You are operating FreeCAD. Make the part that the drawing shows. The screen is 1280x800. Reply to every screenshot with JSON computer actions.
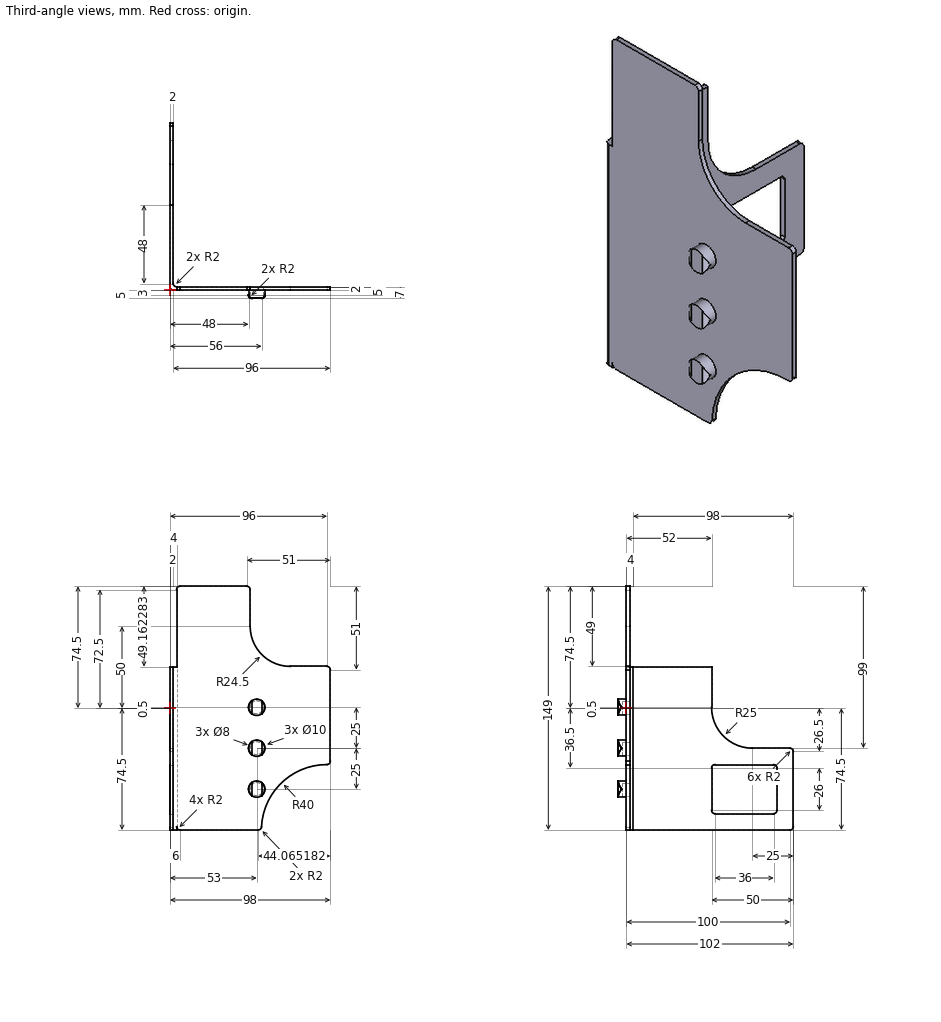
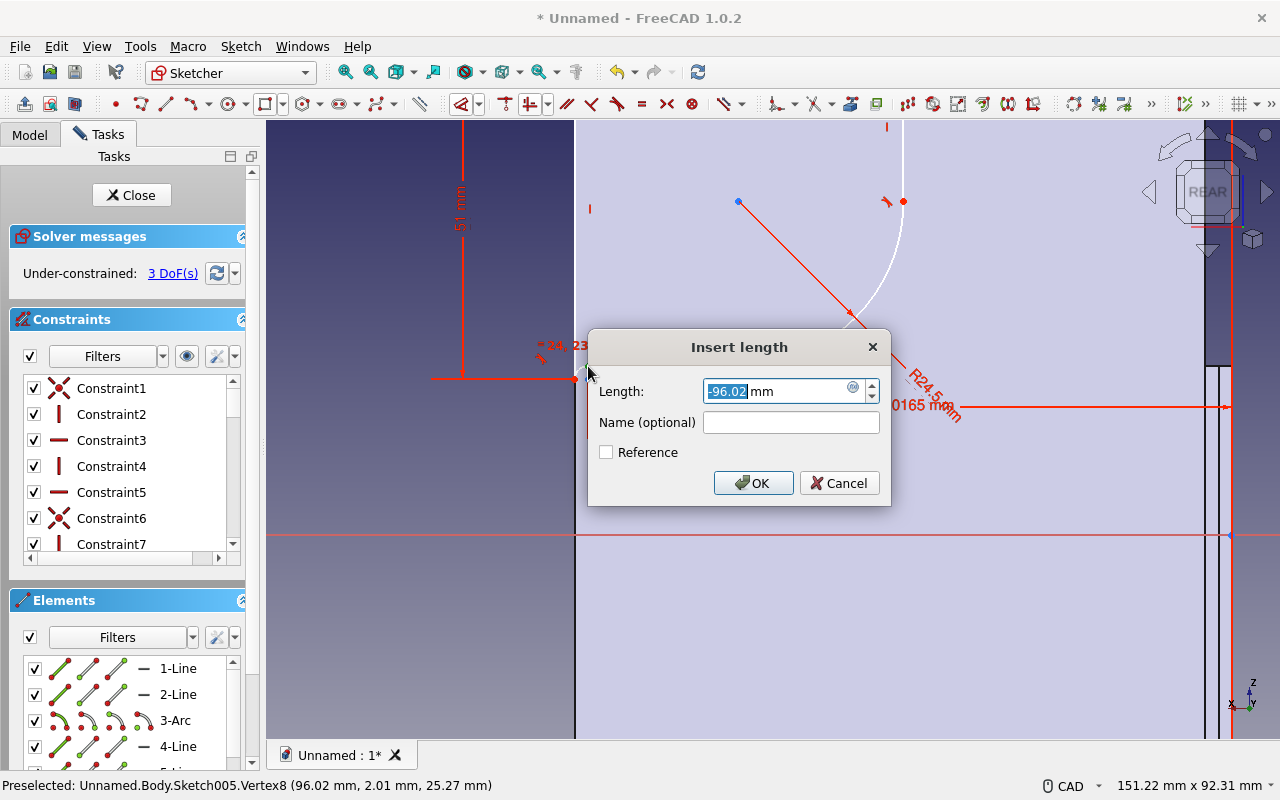
{"action": "type", "text": "-96"}
{"action": "key", "text": "Return"}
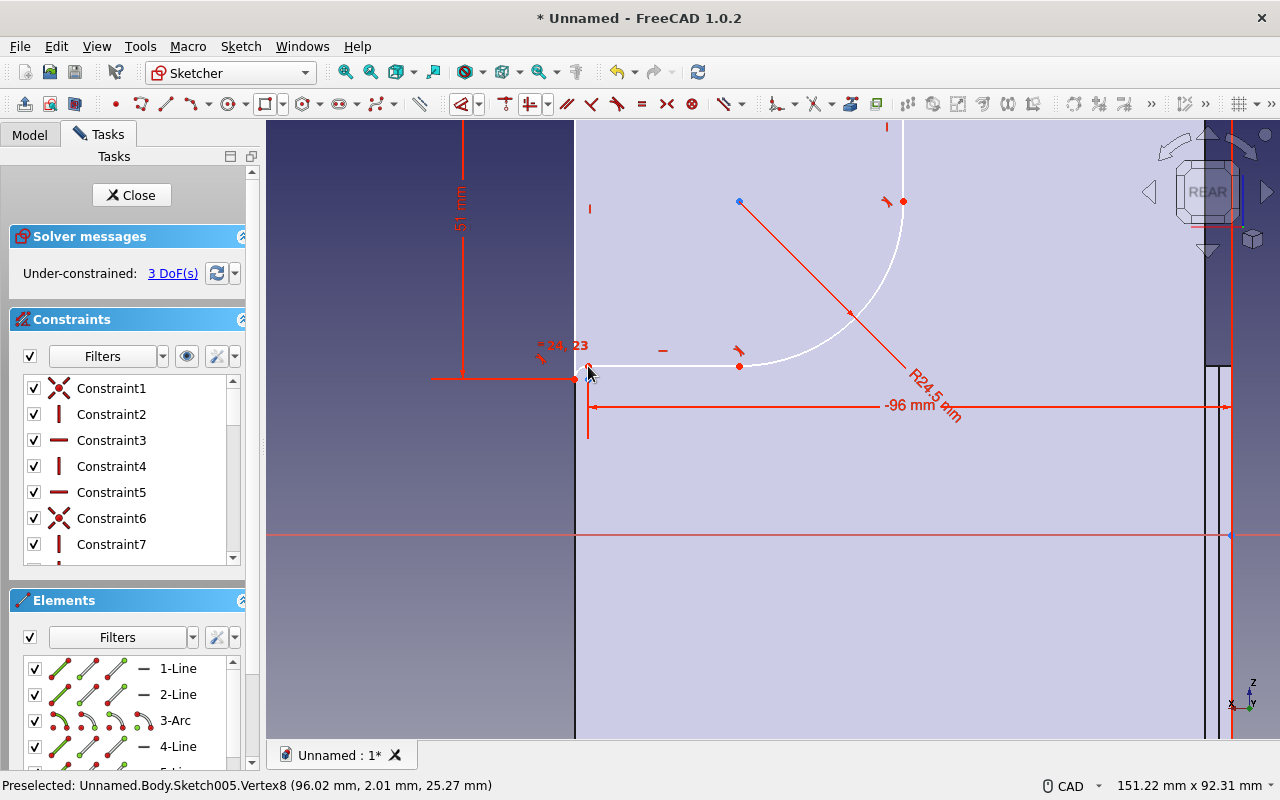
{"action": "left_click", "coordinate": [903, 202]}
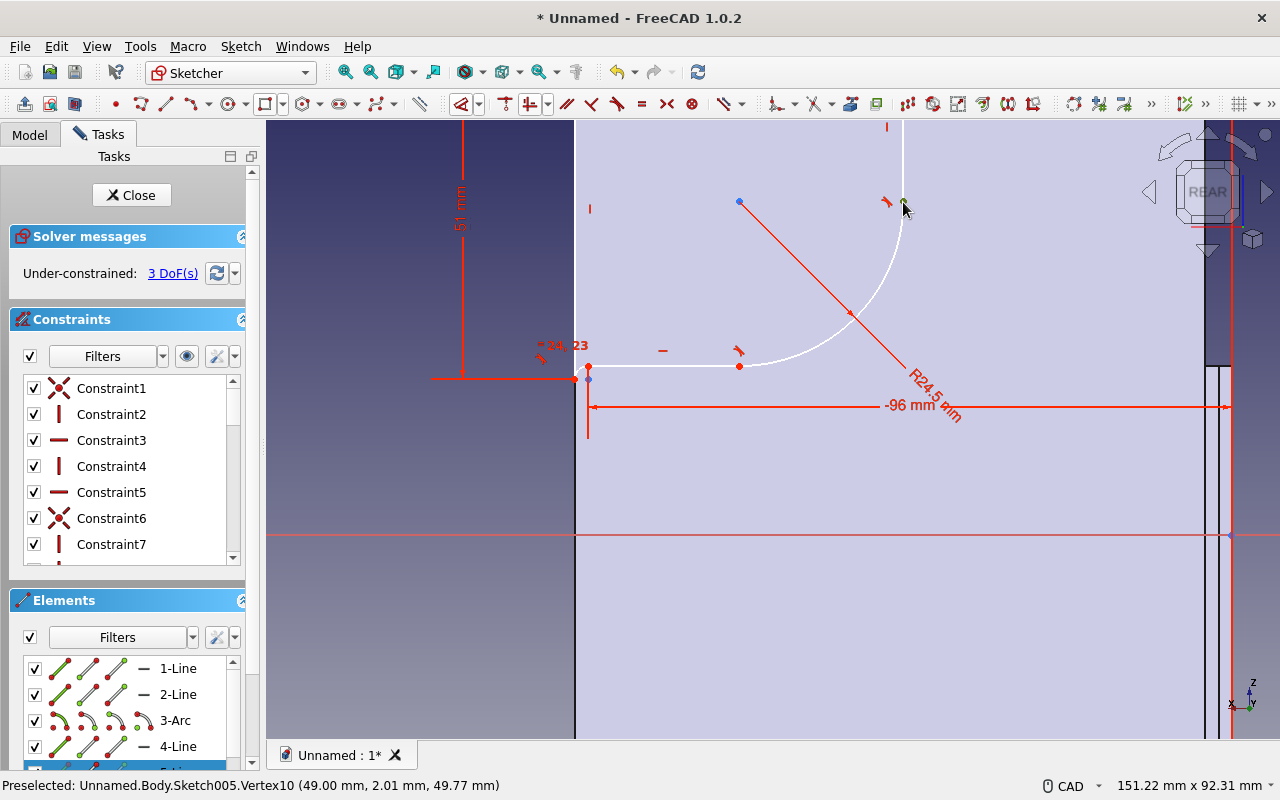
{"action": "key", "text": "i"}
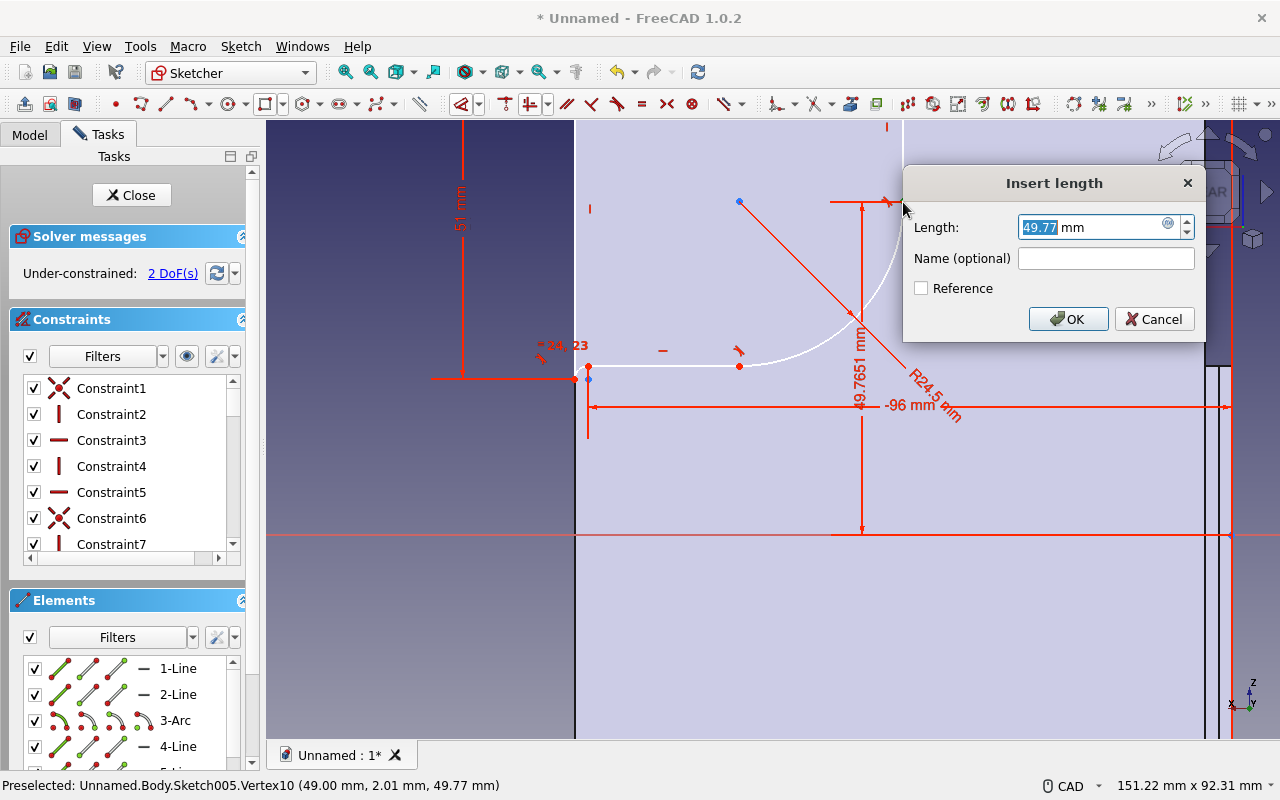
{"action": "type", "text": "50"}
{"action": "key", "text": "Return"}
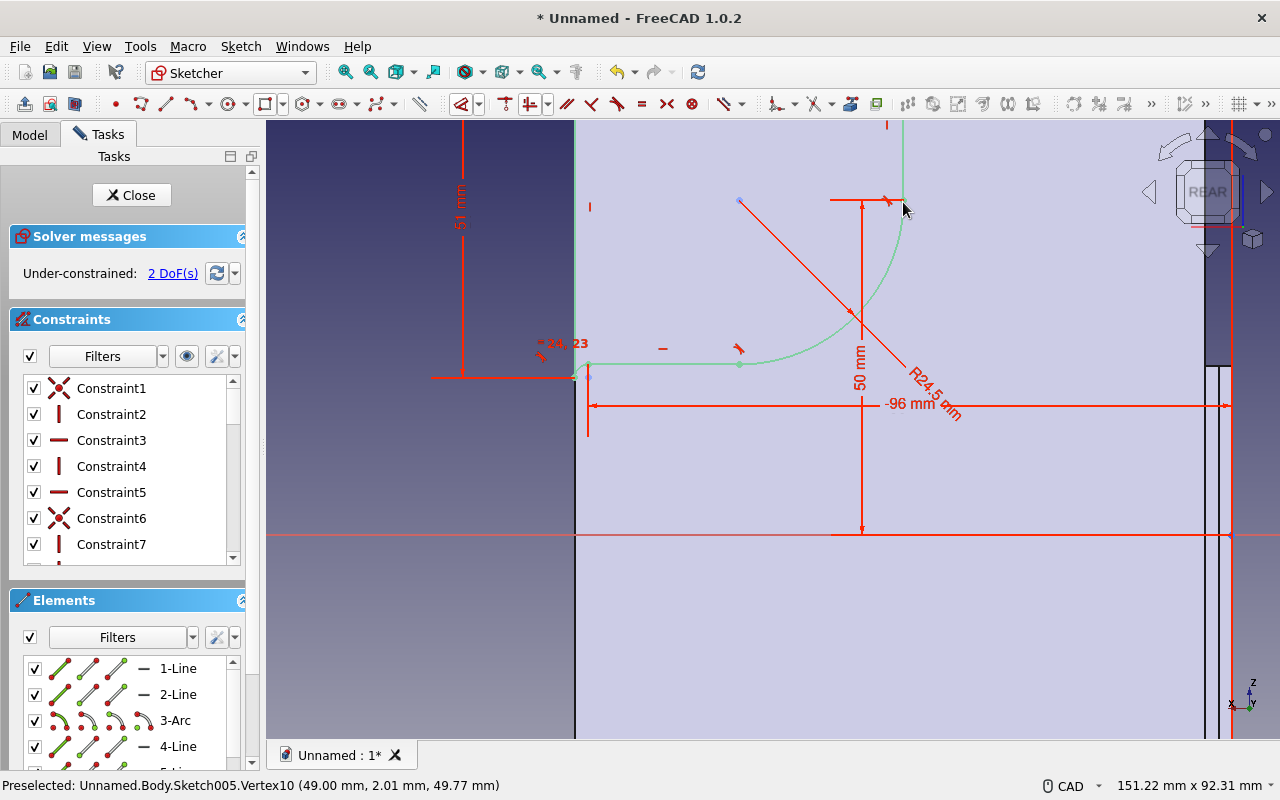
{"action": "scroll", "coordinate": [589, 368], "scroll_direction": "down", "scroll_amount": 5}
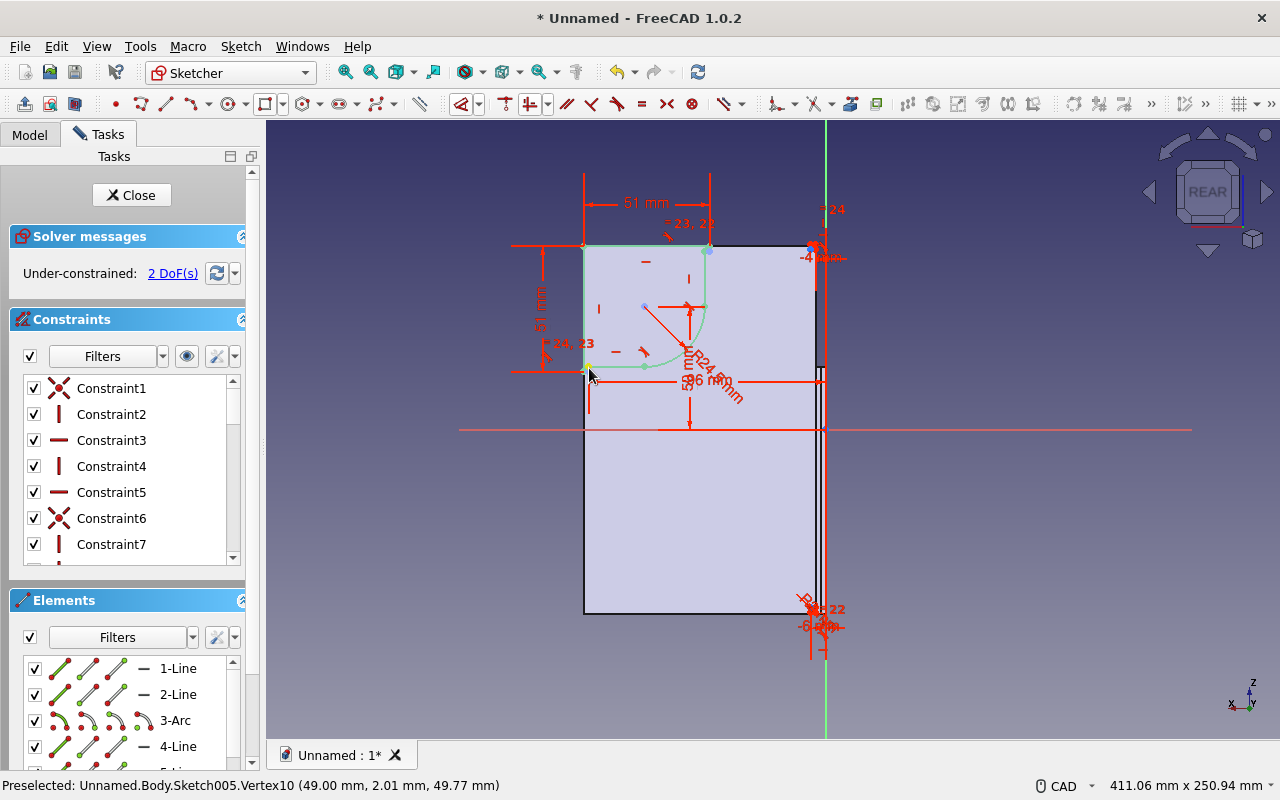
{"action": "scroll", "coordinate": [811, 613], "scroll_direction": "up", "scroll_amount": 5}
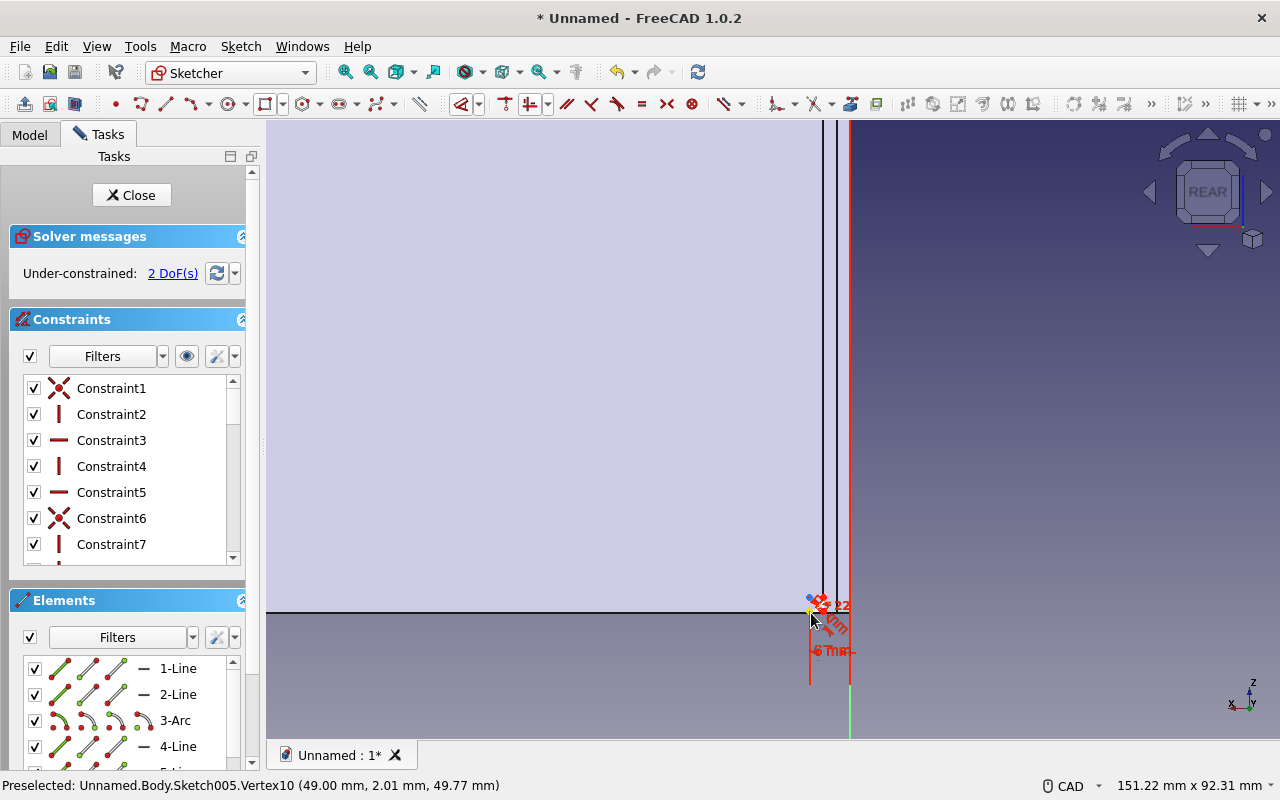
{"action": "left_click", "coordinate": [810, 611]}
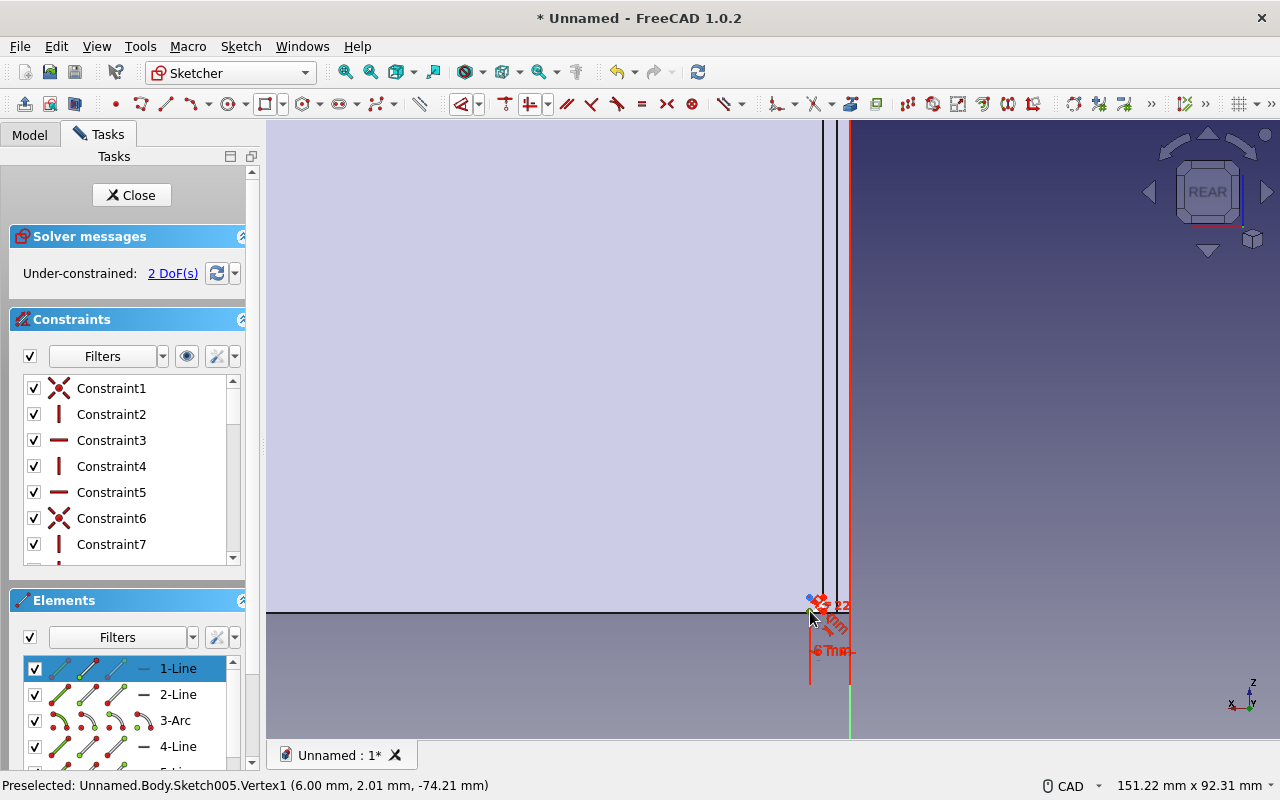
{"action": "left_click", "coordinate": [478, 104]}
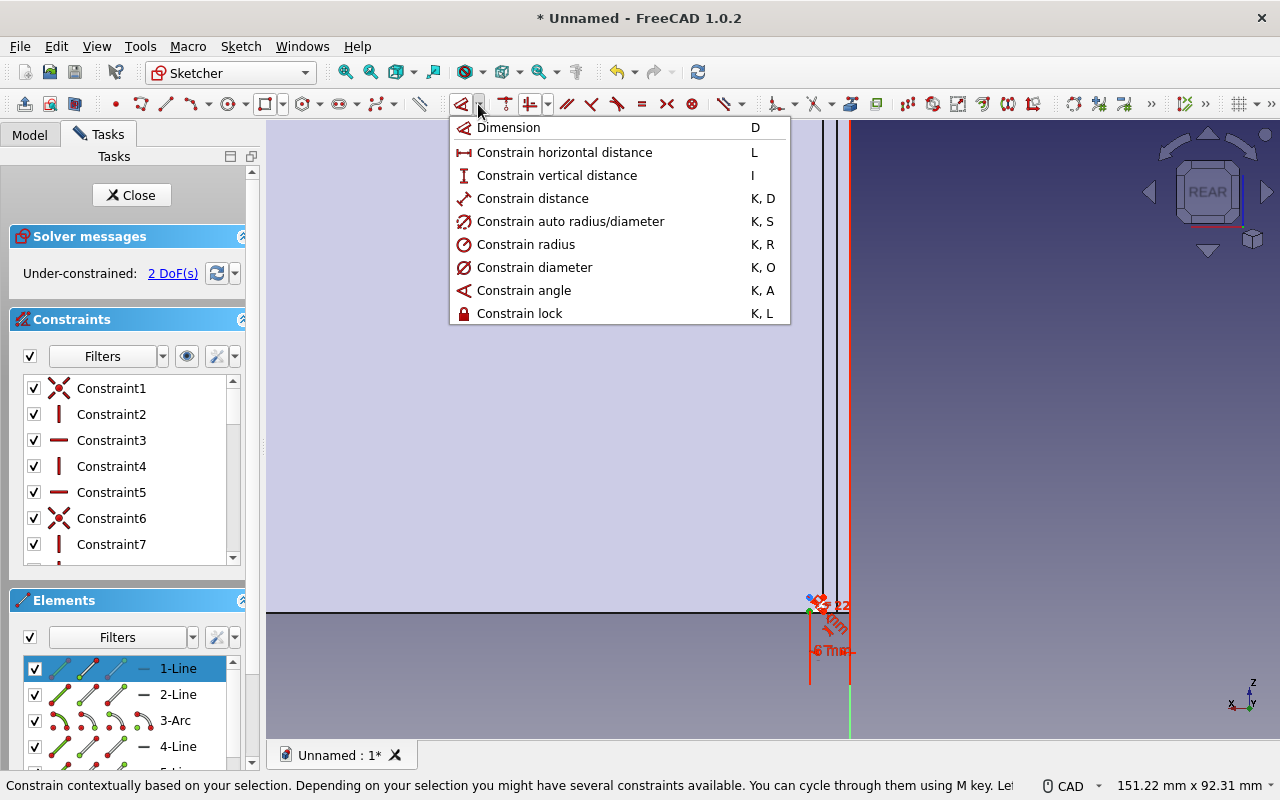
{"action": "left_click", "coordinate": [620, 176]}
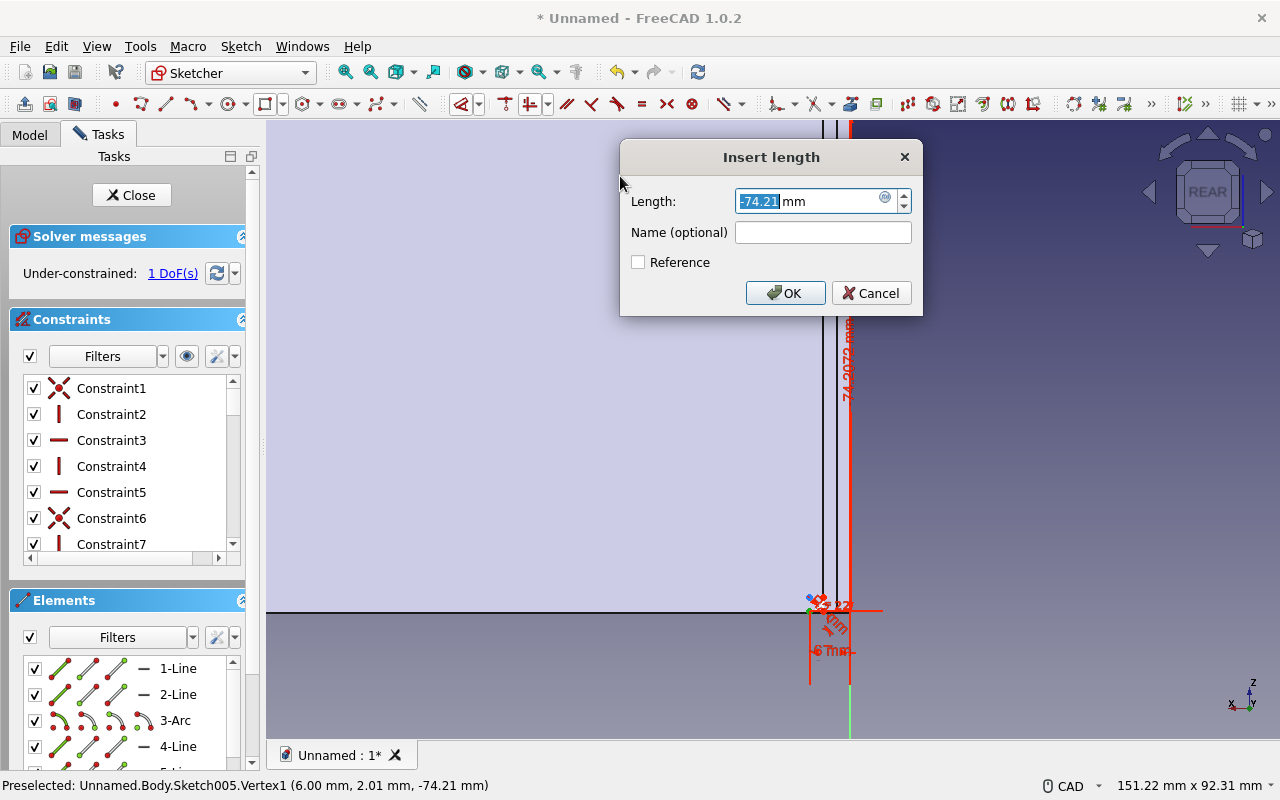
{"action": "type", "text": "-74.5"}
{"action": "key", "text": "Return"}